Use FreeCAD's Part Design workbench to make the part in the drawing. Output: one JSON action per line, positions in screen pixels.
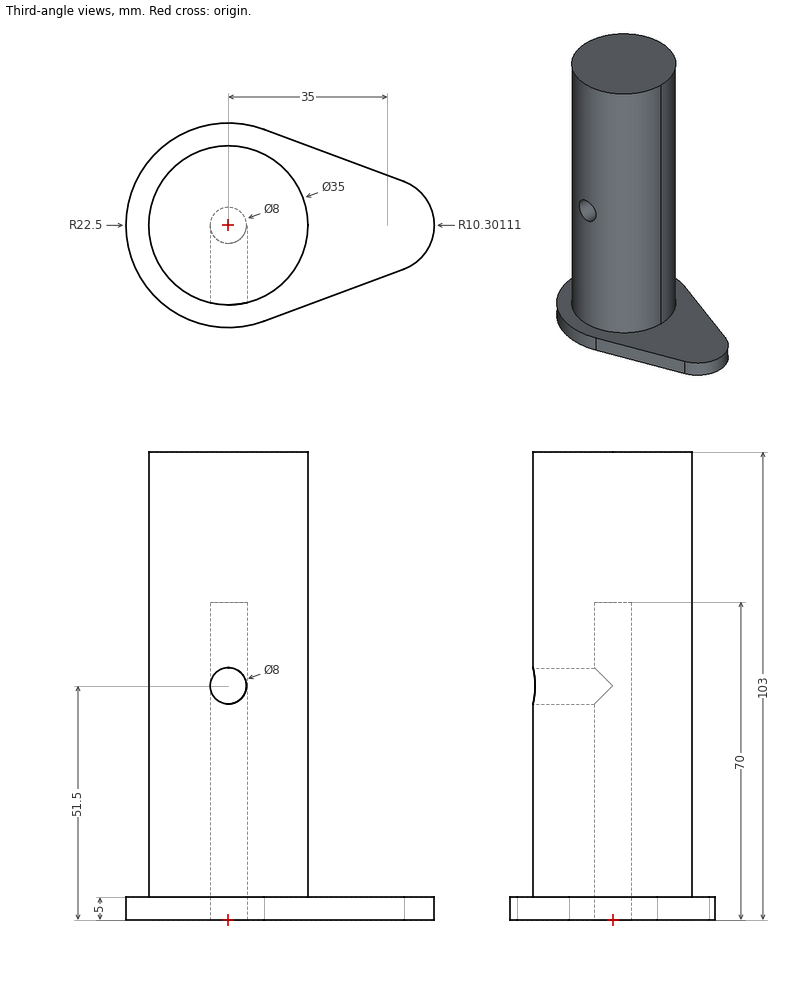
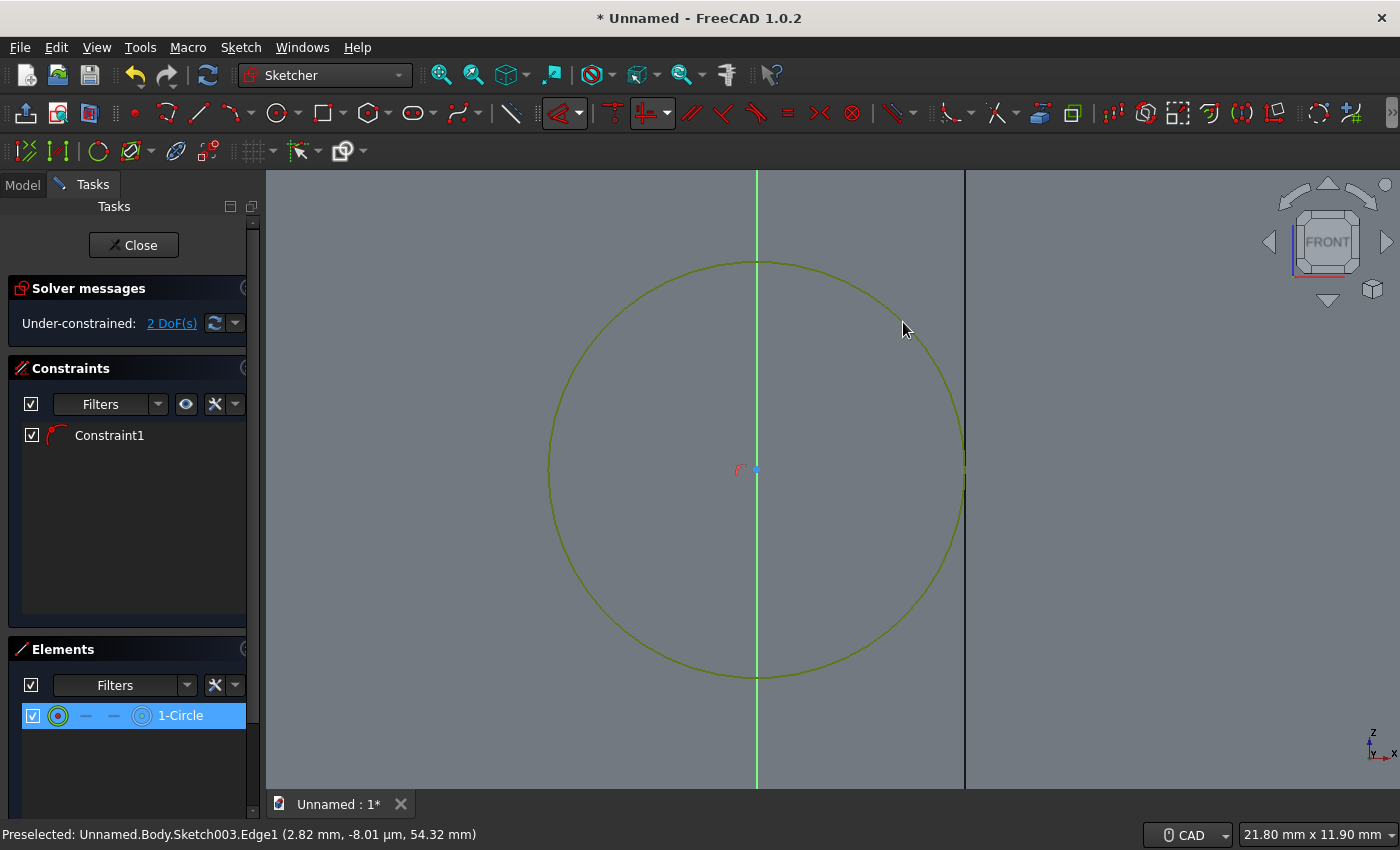
{"action": "key", "text": "k o"}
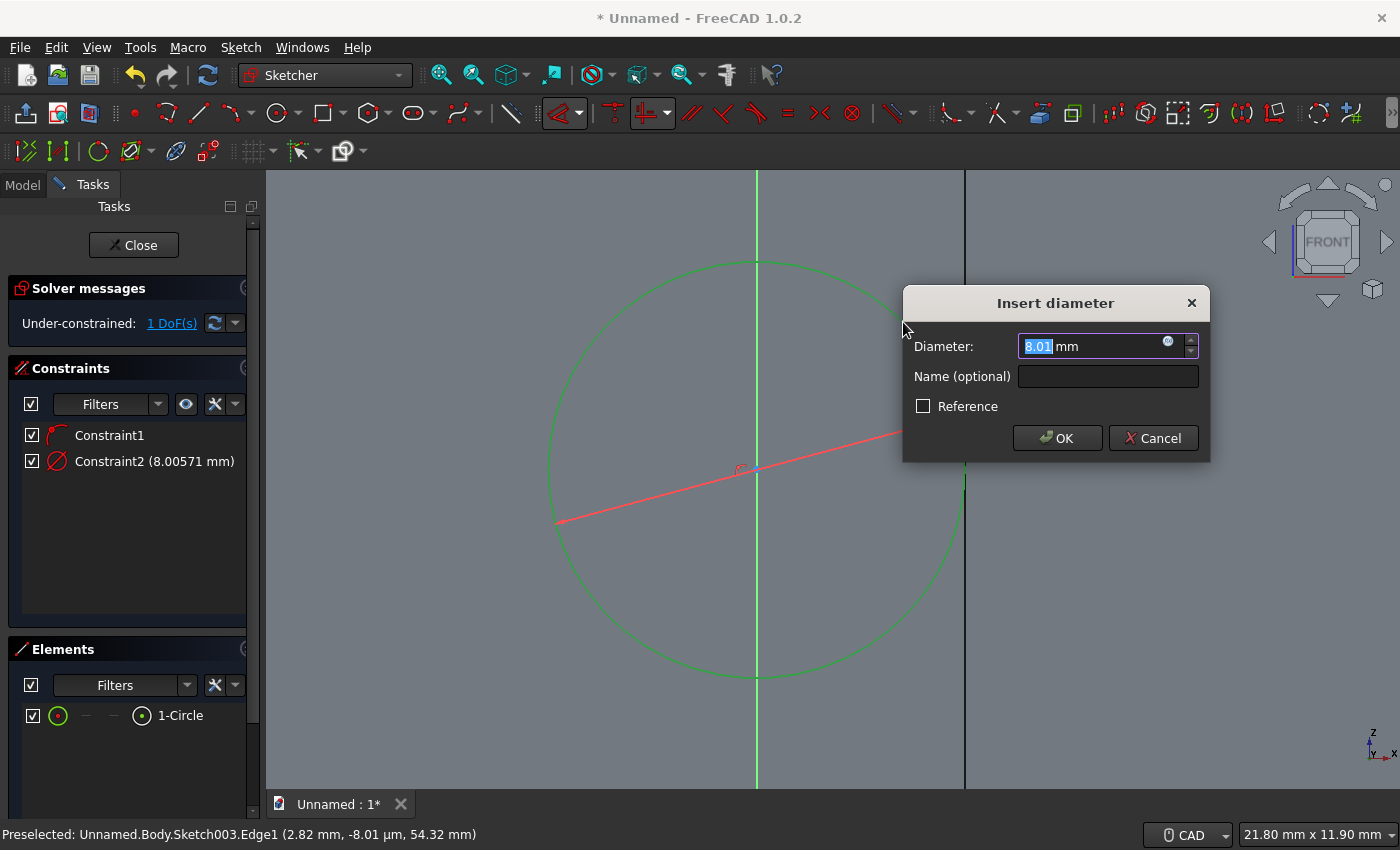
{"action": "type", "text": "8"}
{"action": "key", "text": "Return"}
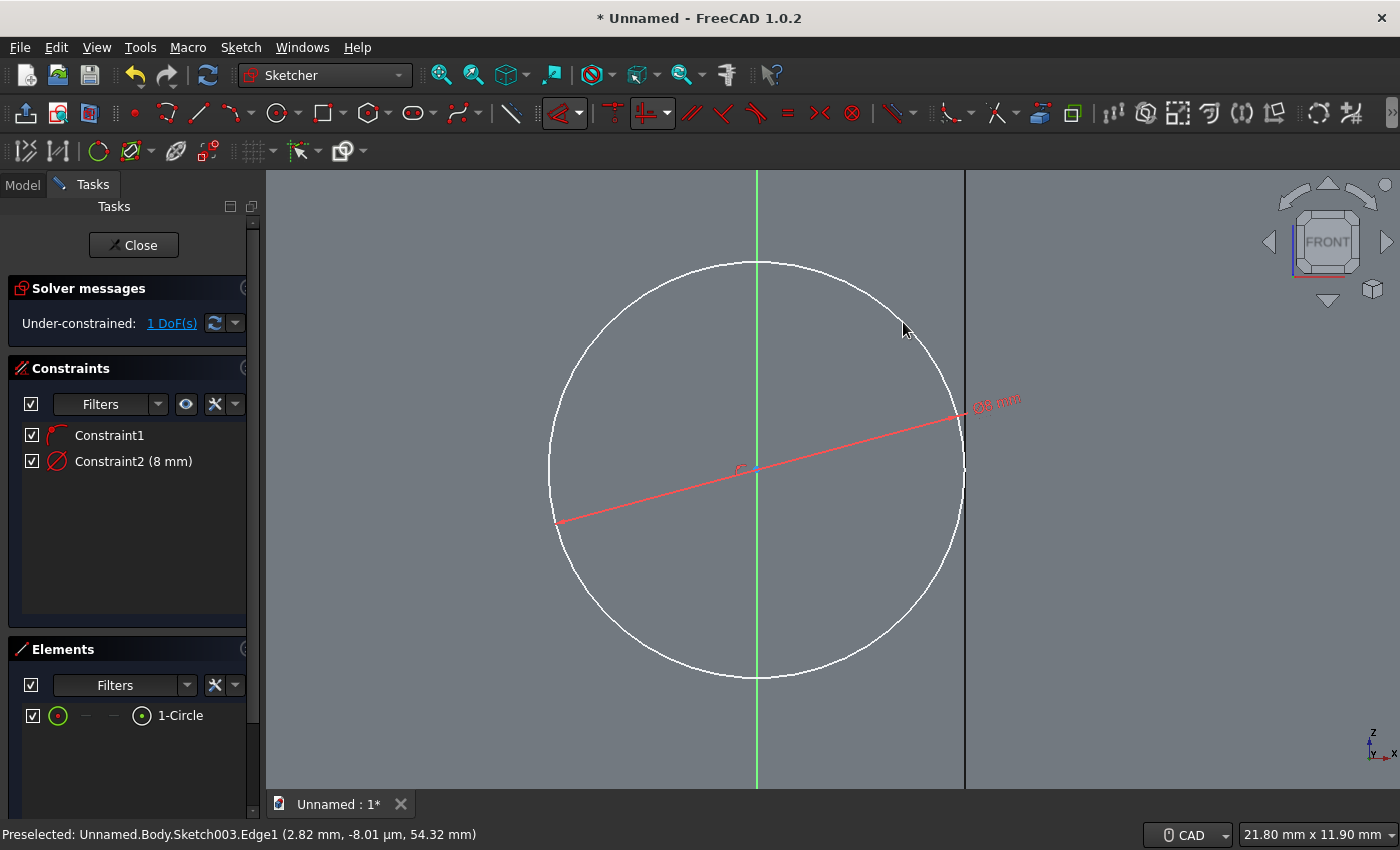
{"action": "left_click", "coordinate": [757, 470]}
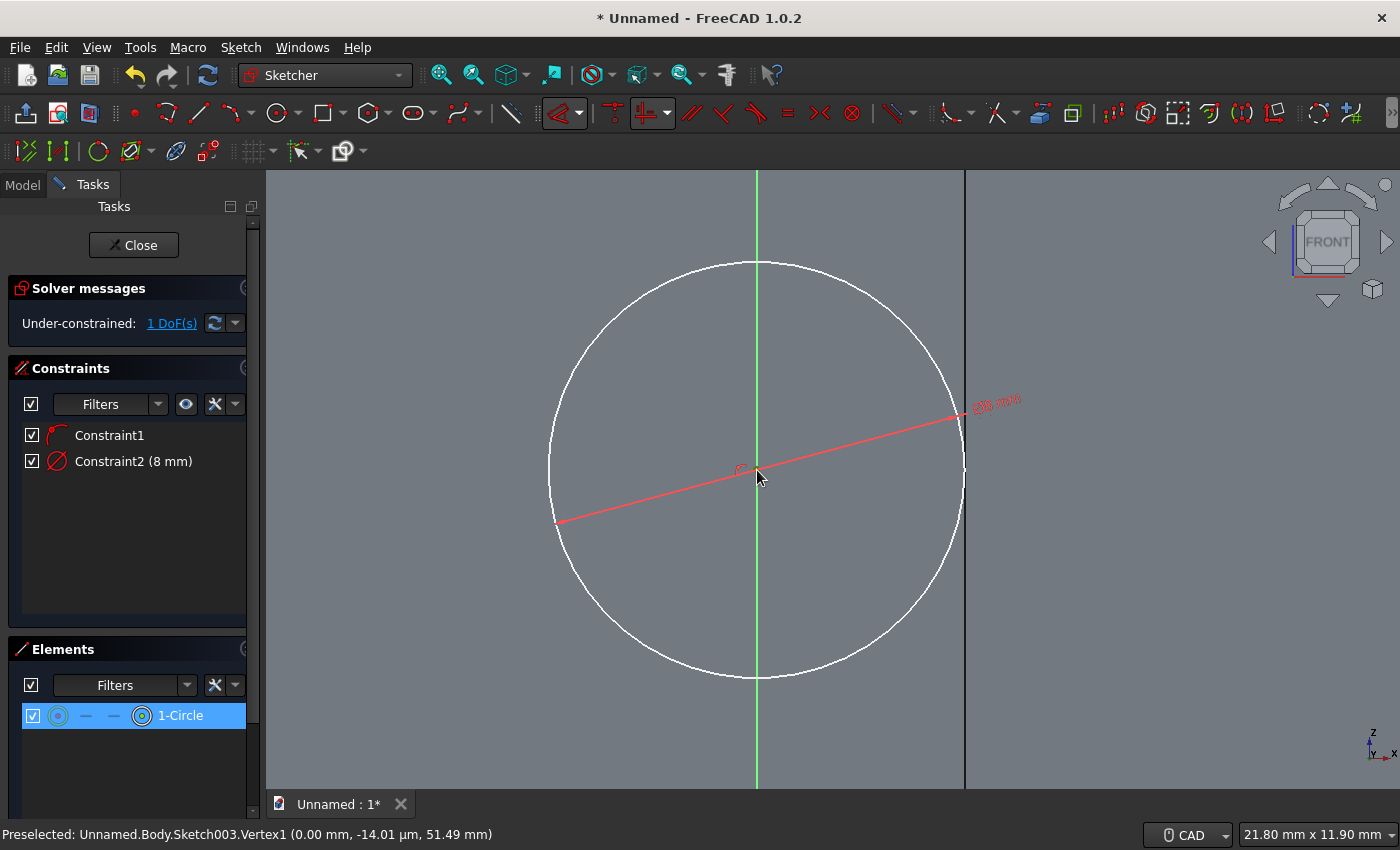
{"action": "left_click", "coordinate": [582, 114]}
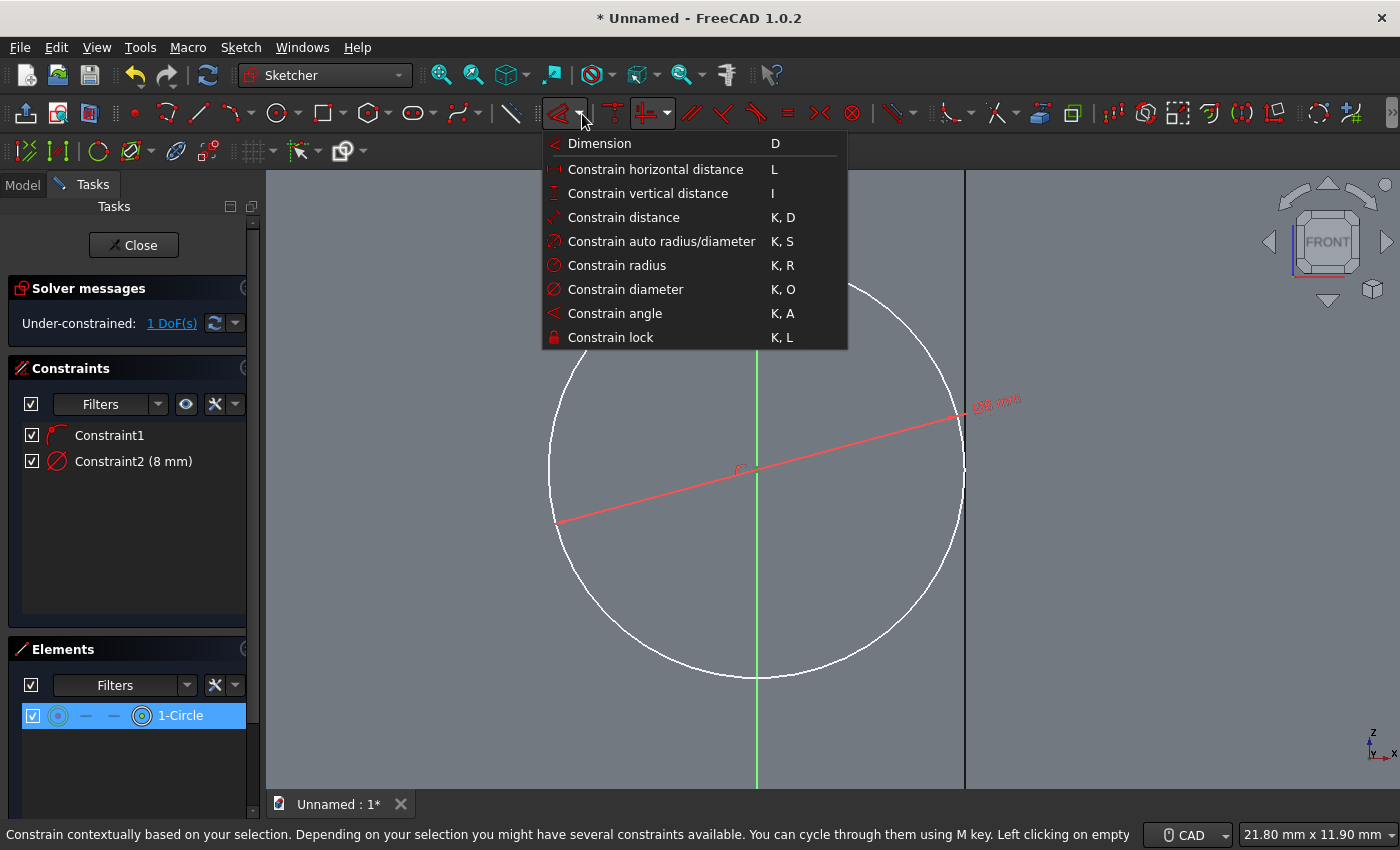
{"action": "left_click", "coordinate": [695, 193]}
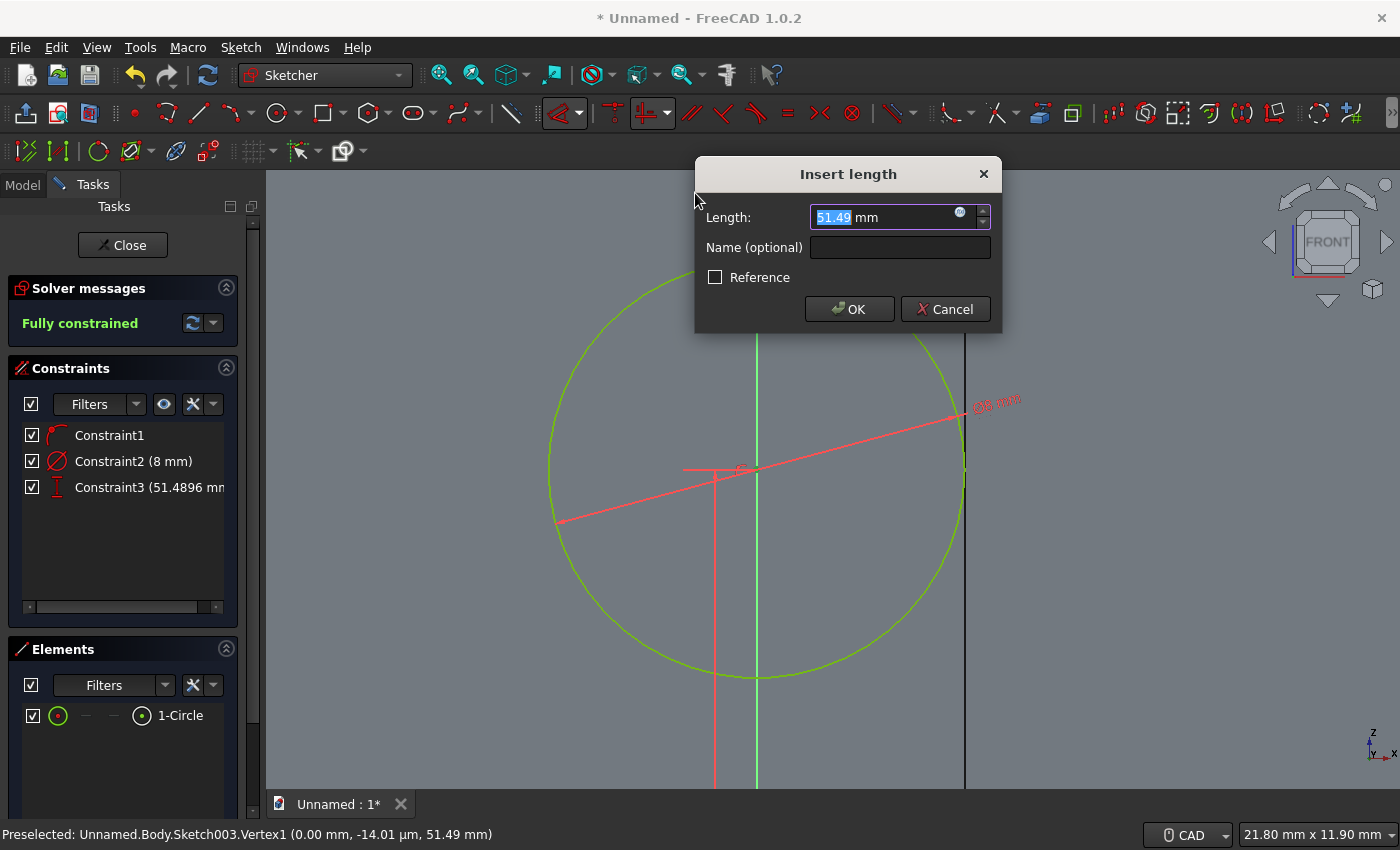
{"action": "type", "text": "51.5"}
{"action": "key", "text": "Return"}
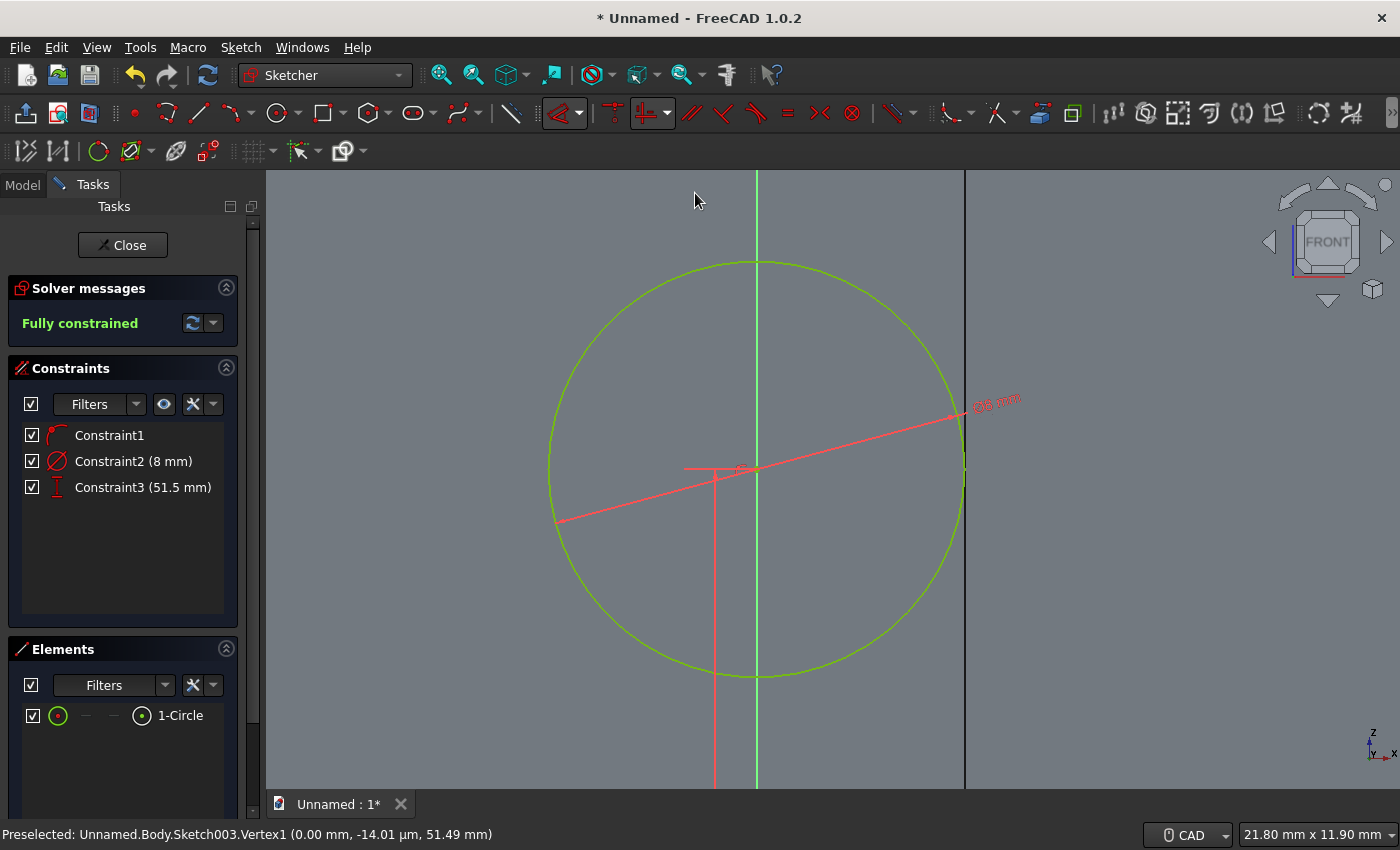
{"action": "left_click", "coordinate": [123, 245]}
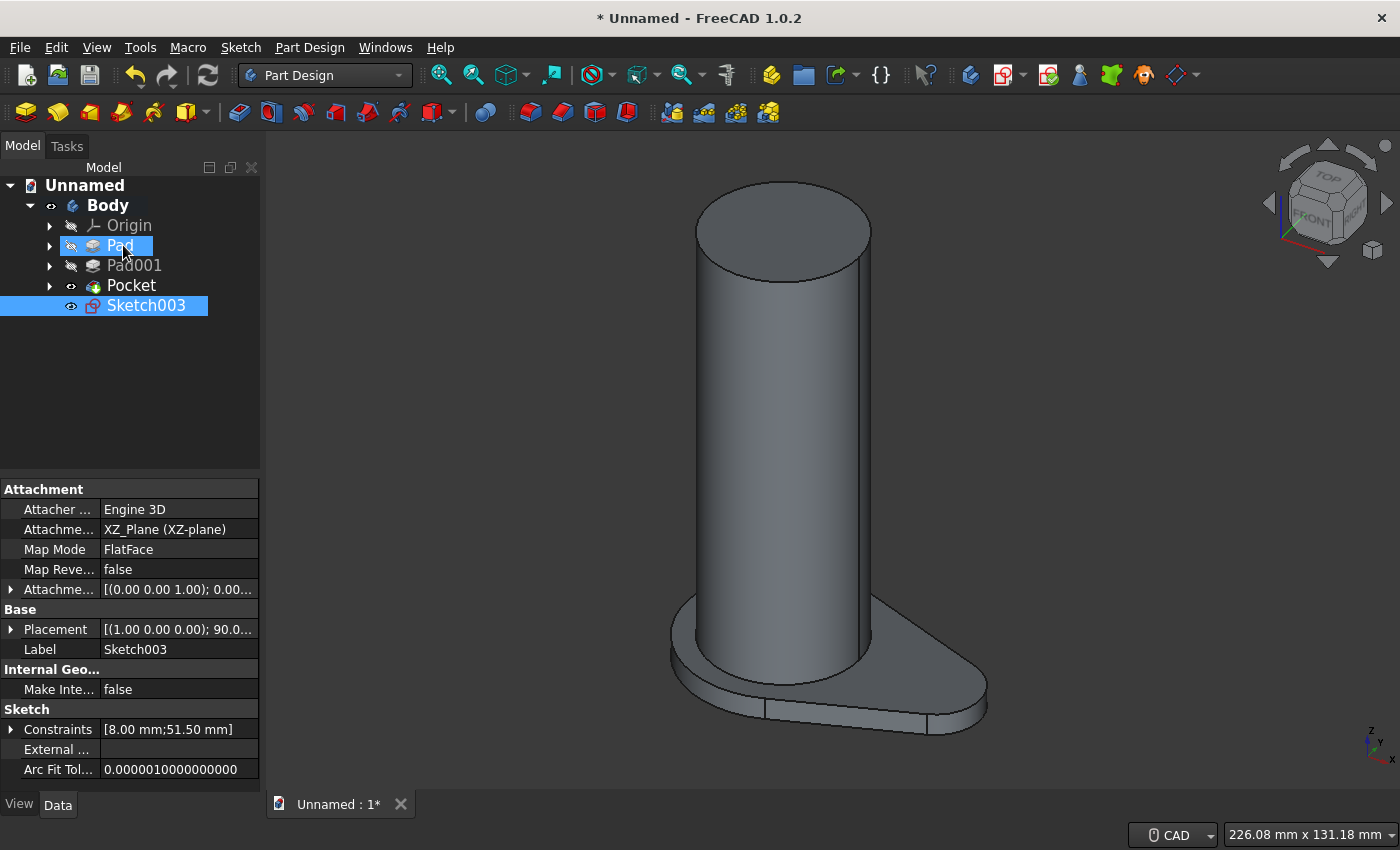
{"action": "left_click", "coordinate": [240, 112]}